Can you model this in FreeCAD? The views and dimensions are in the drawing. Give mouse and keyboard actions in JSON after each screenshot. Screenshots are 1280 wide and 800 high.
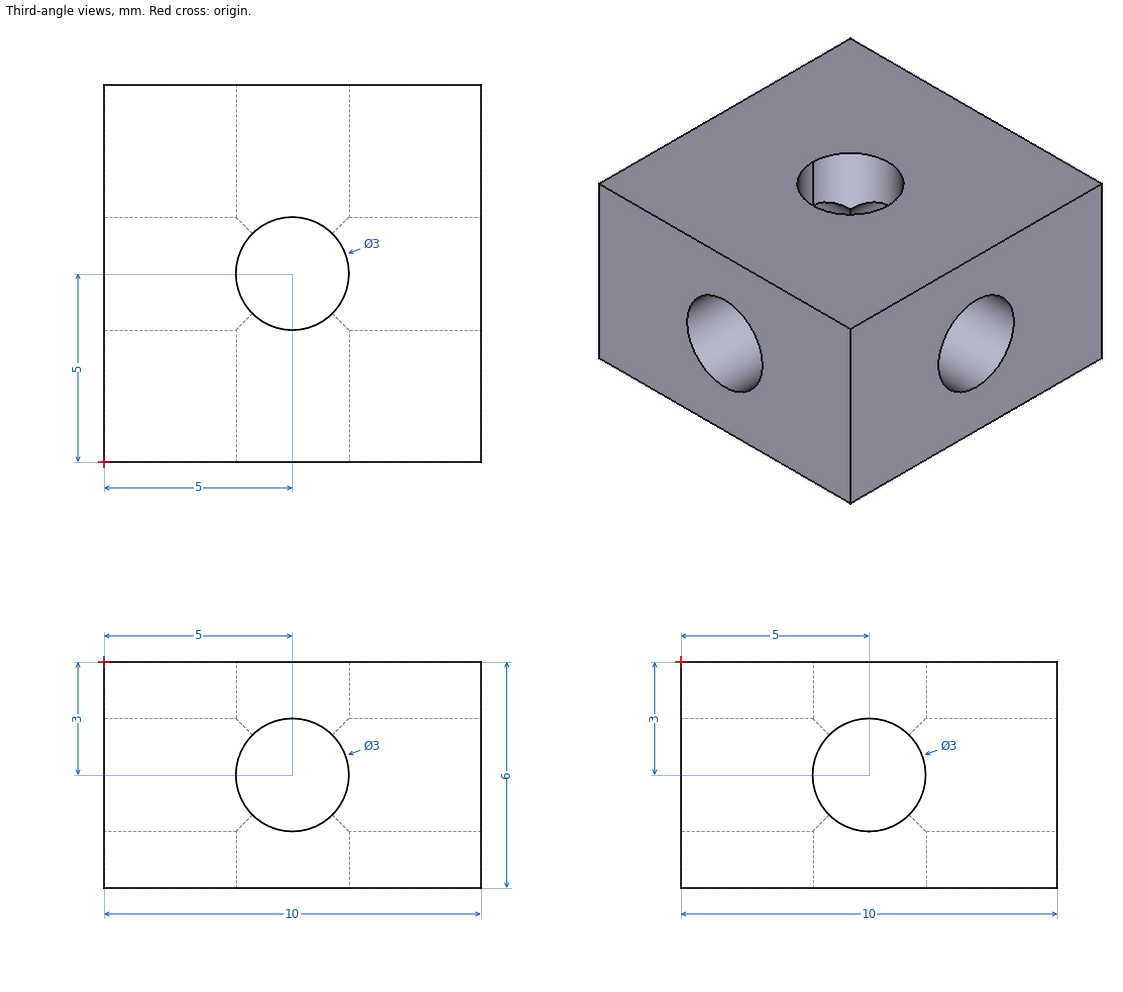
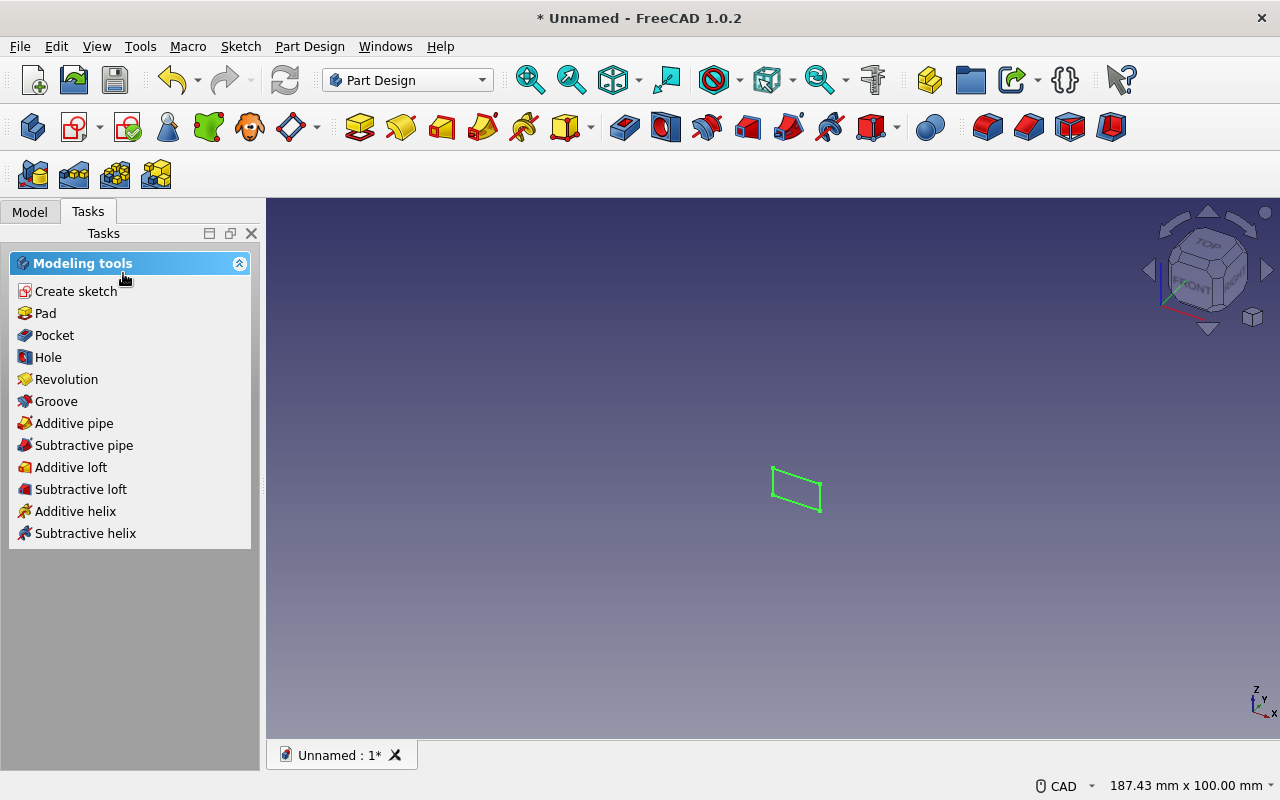
{"action": "left_click", "coordinate": [360, 128]}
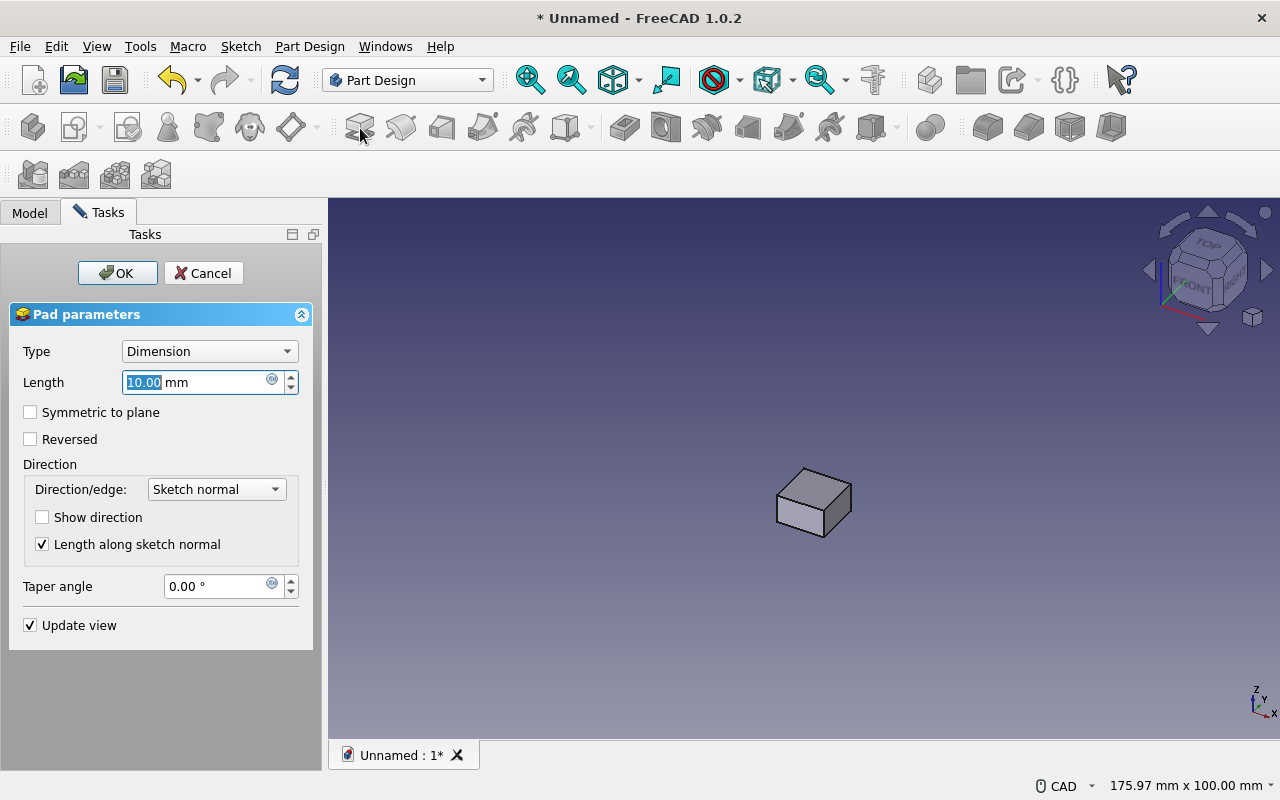
{"action": "type", "text": "10"}
{"action": "key", "text": "Tab"}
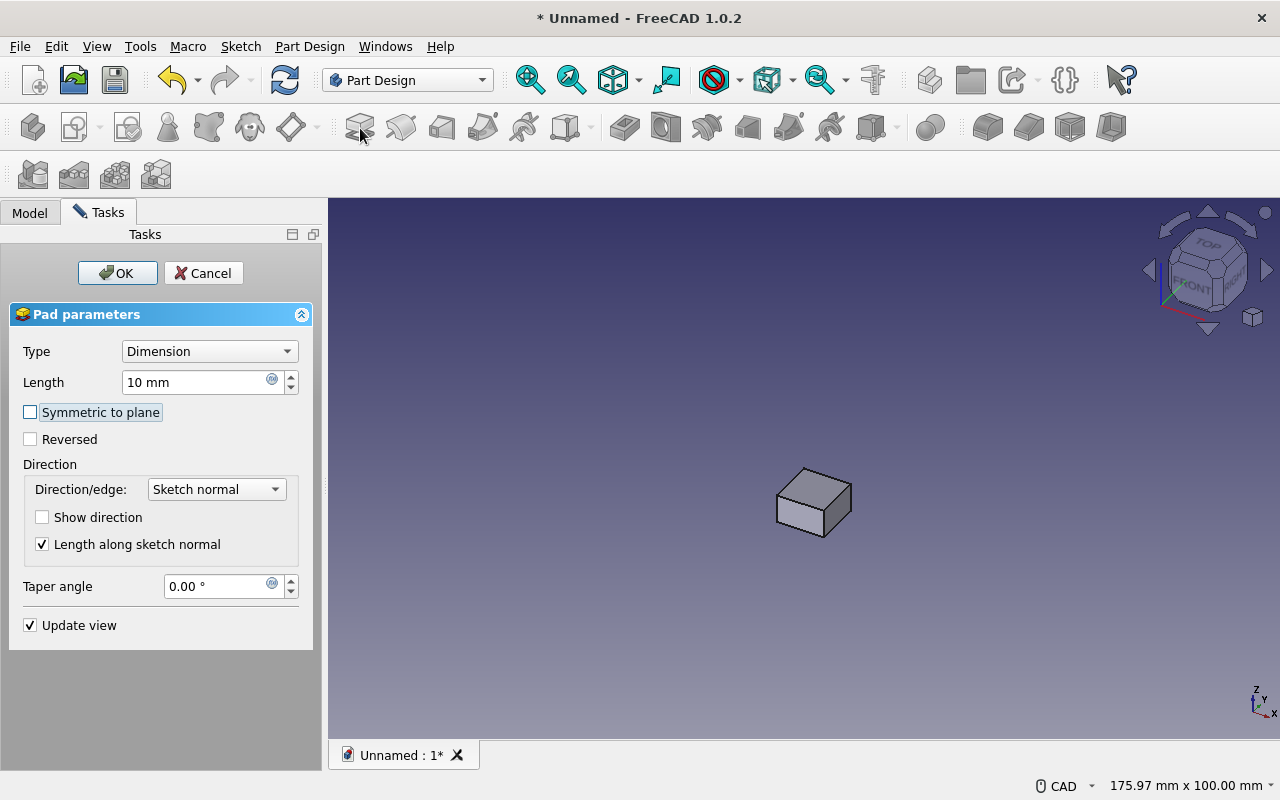
{"action": "left_click", "coordinate": [31, 439]}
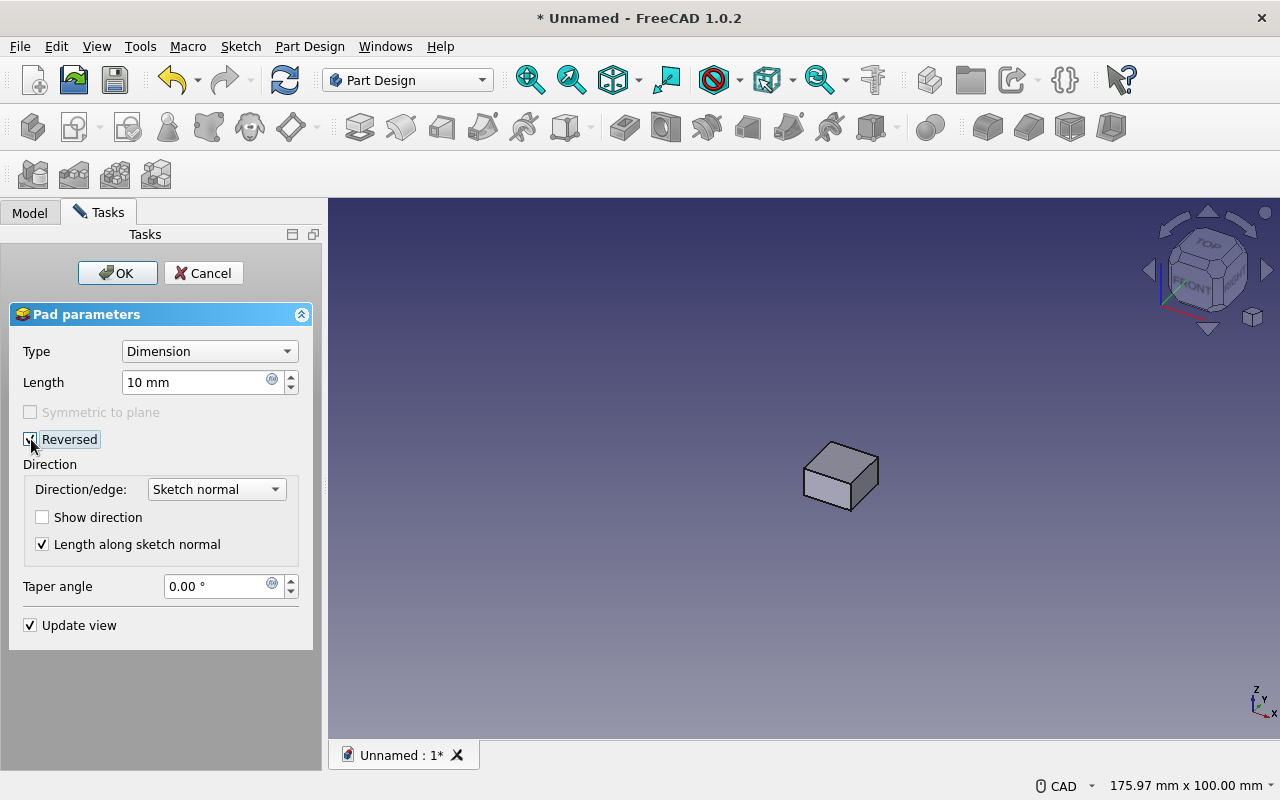
{"action": "left_click", "coordinate": [118, 273]}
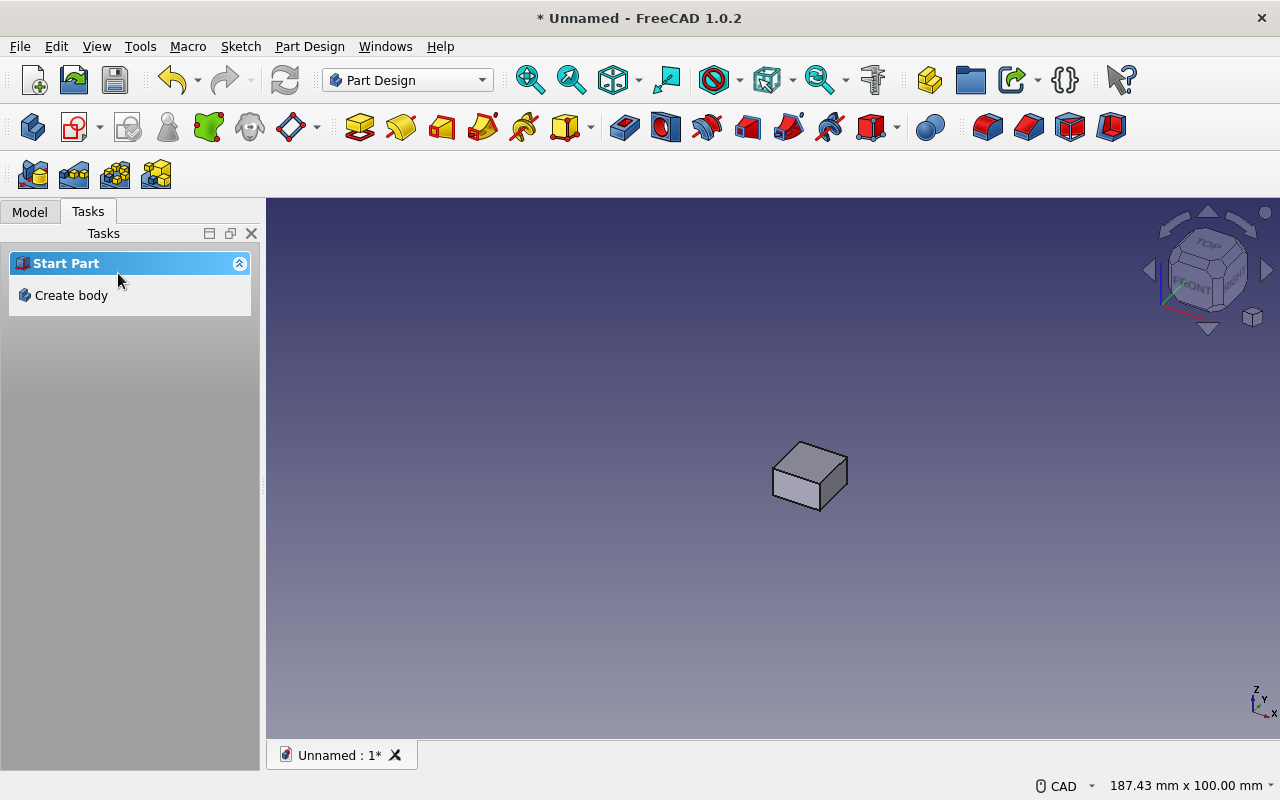
{"action": "left_click", "coordinate": [531, 80]}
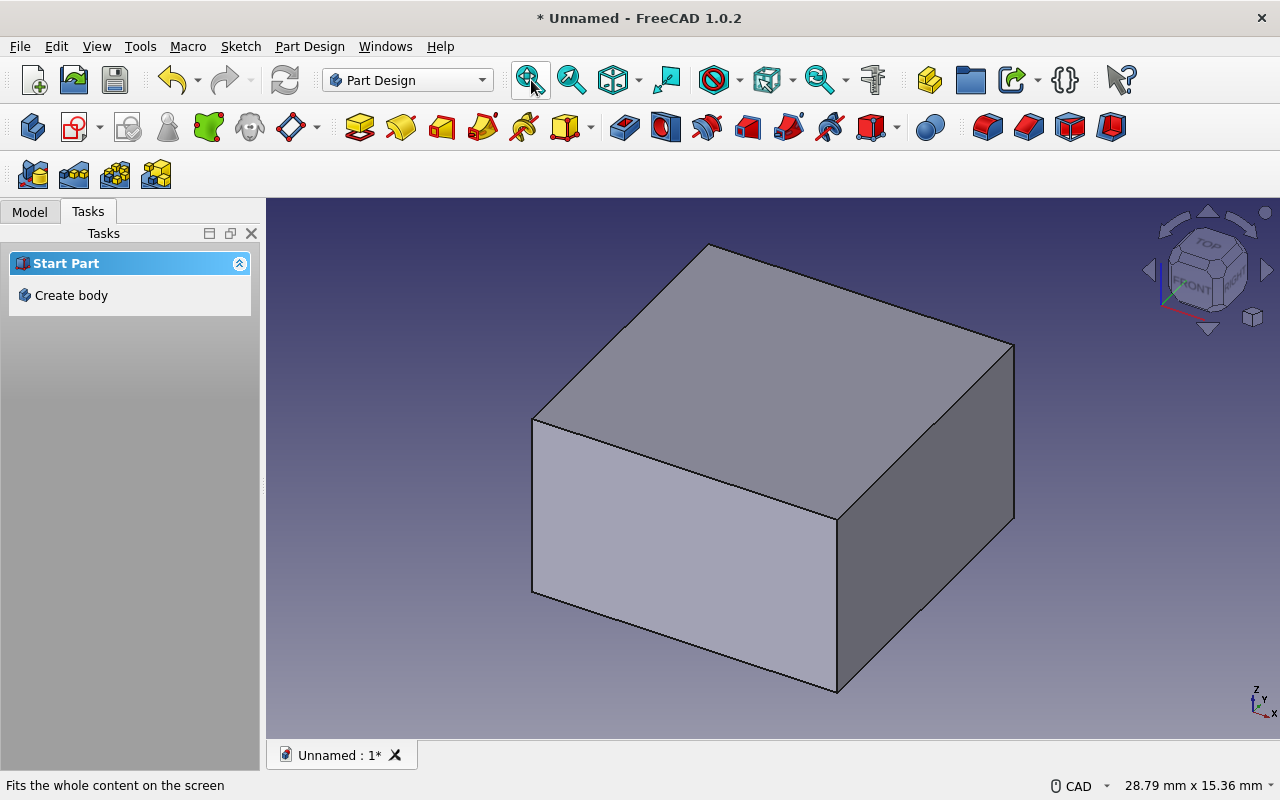
{"action": "left_click", "coordinate": [773, 381]}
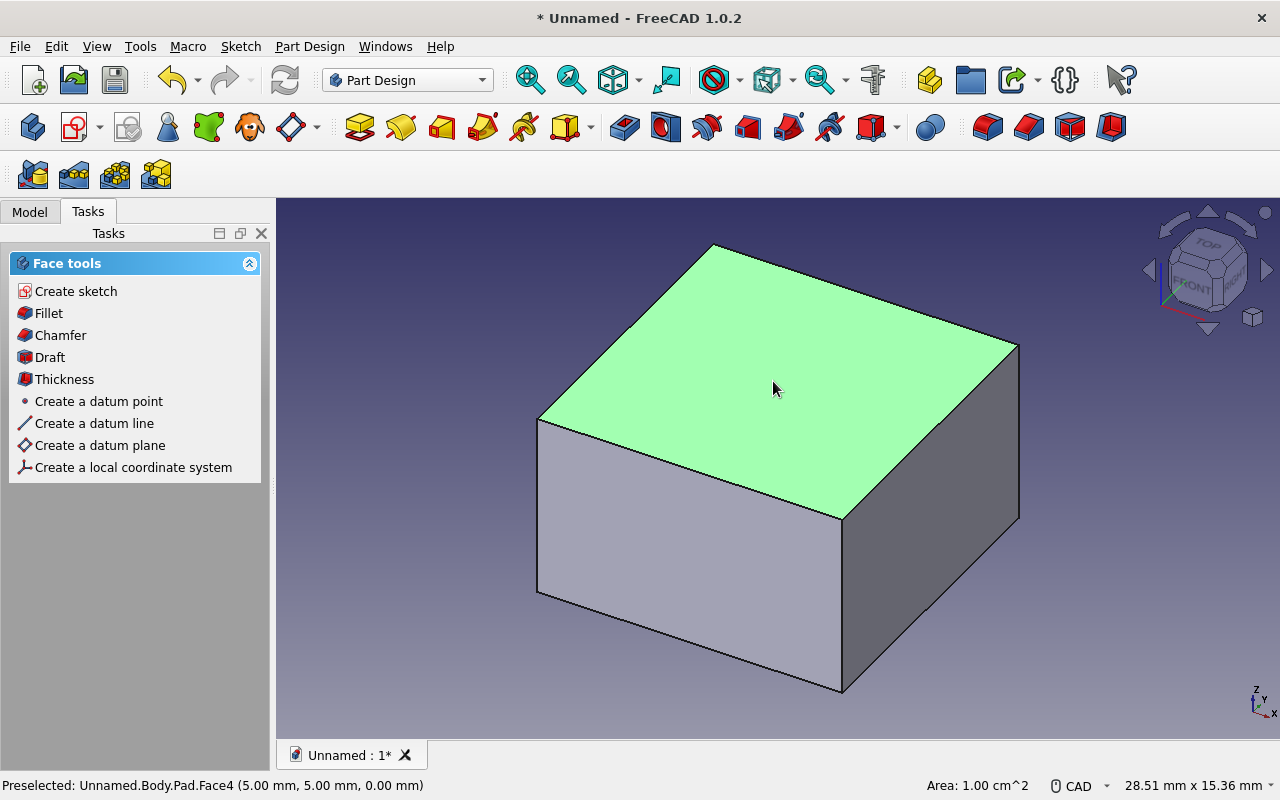
{"action": "left_click", "coordinate": [74, 128]}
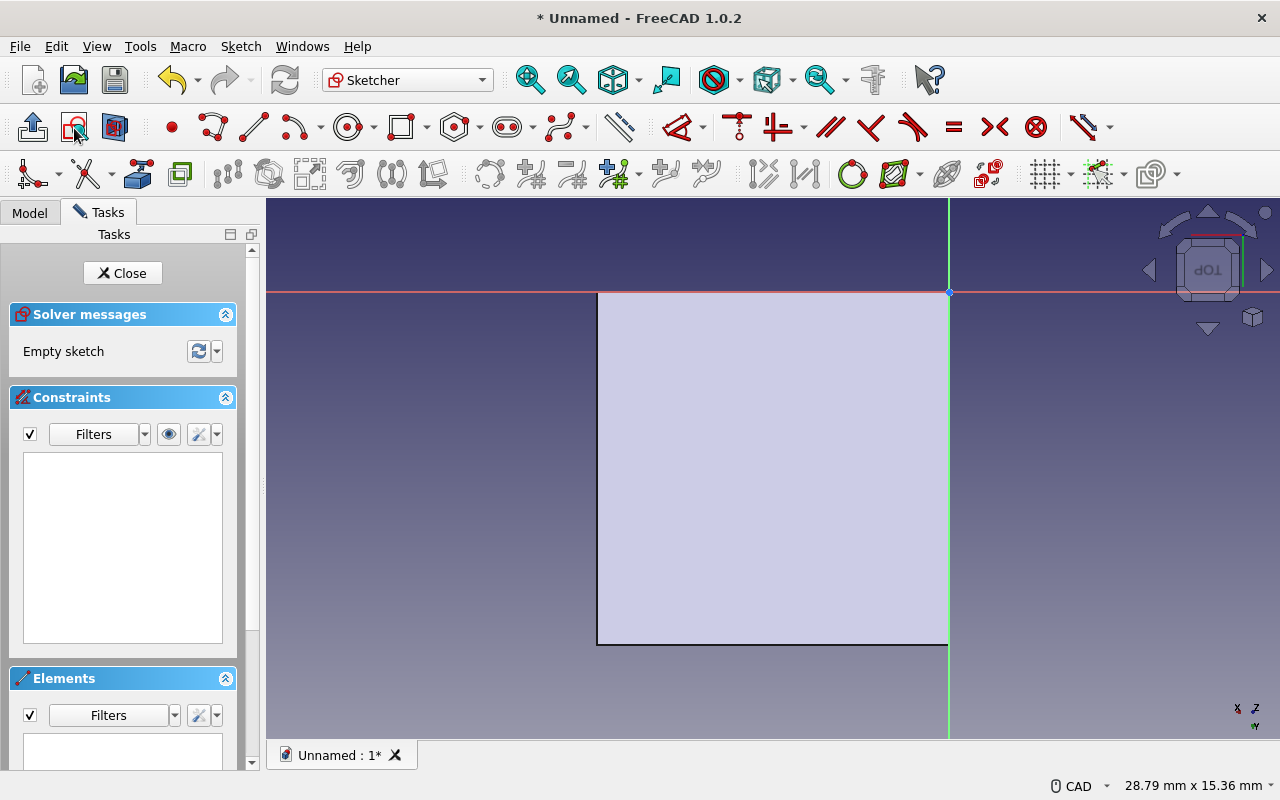
{"action": "scroll", "coordinate": [1099, 282], "scroll_direction": "up", "scroll_amount": 2}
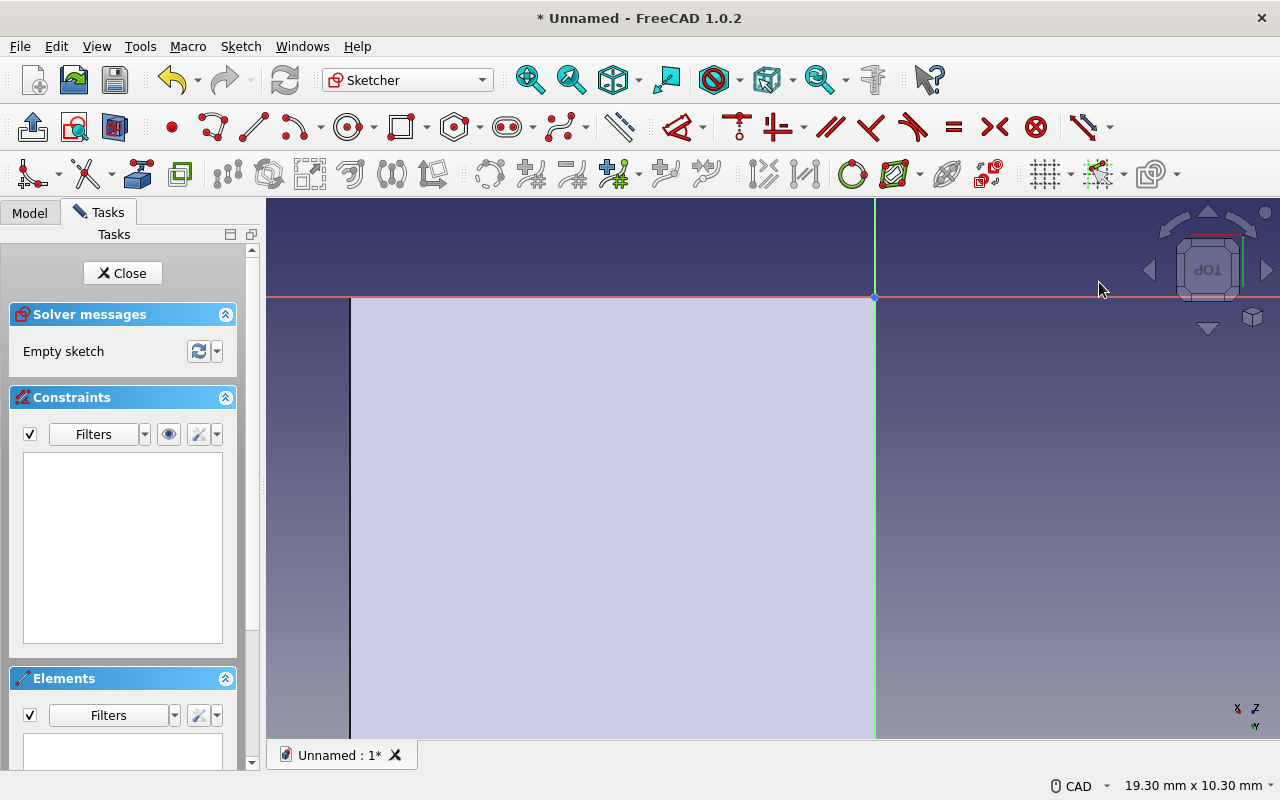
{"action": "left_click", "coordinate": [348, 128]}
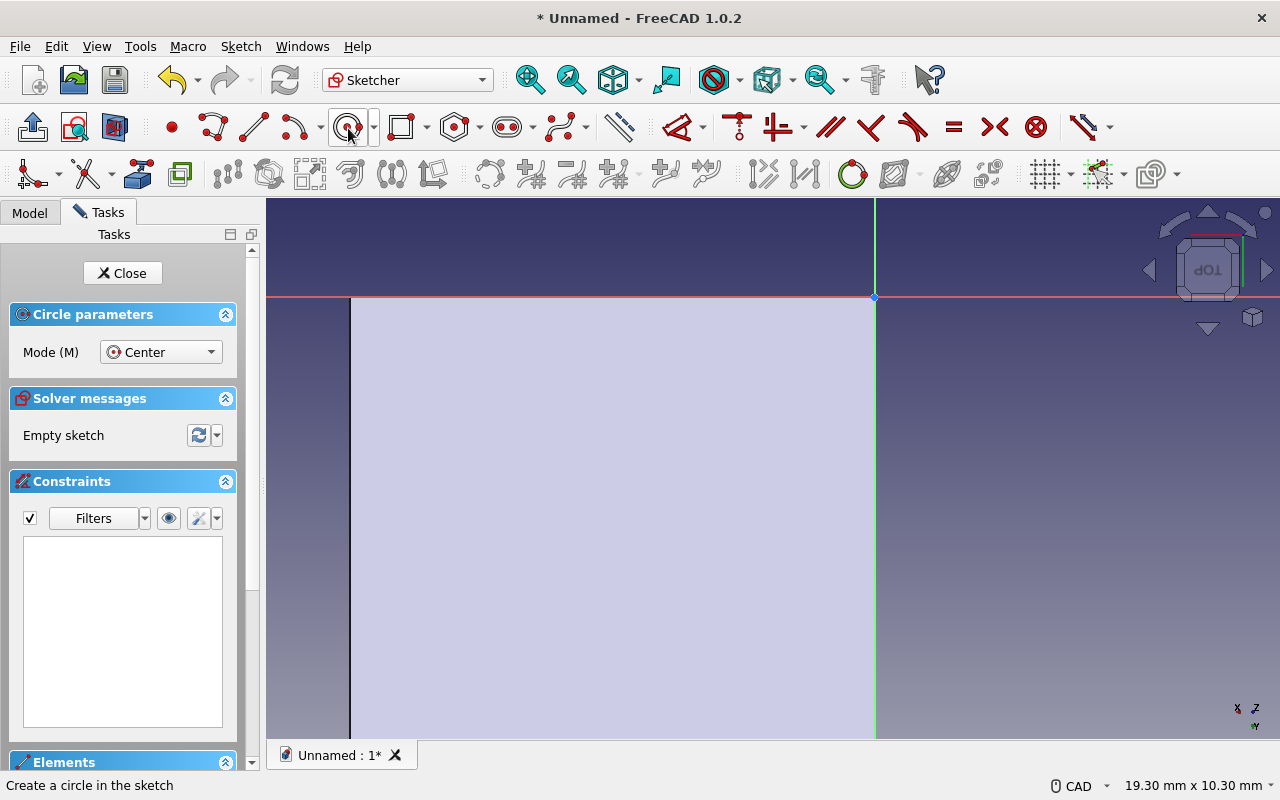
{"action": "left_click", "coordinate": [612, 560]}
{"action": "mouse_move", "coordinate": [668, 504]}